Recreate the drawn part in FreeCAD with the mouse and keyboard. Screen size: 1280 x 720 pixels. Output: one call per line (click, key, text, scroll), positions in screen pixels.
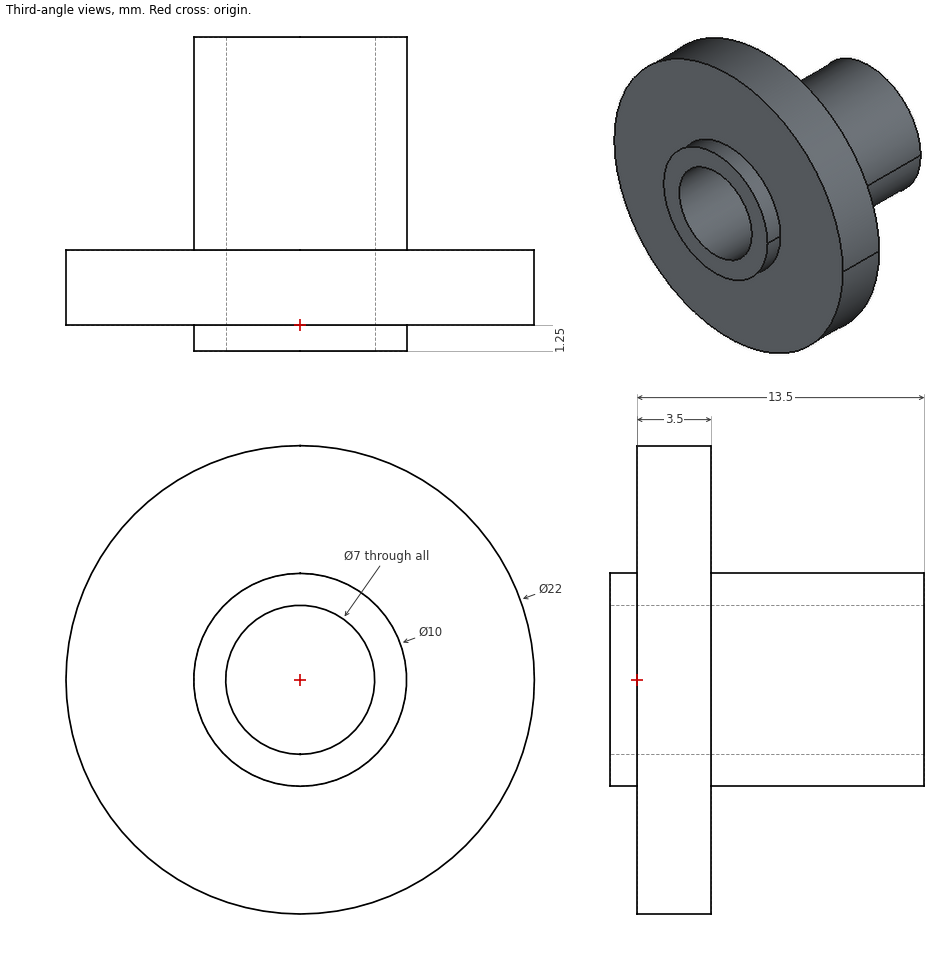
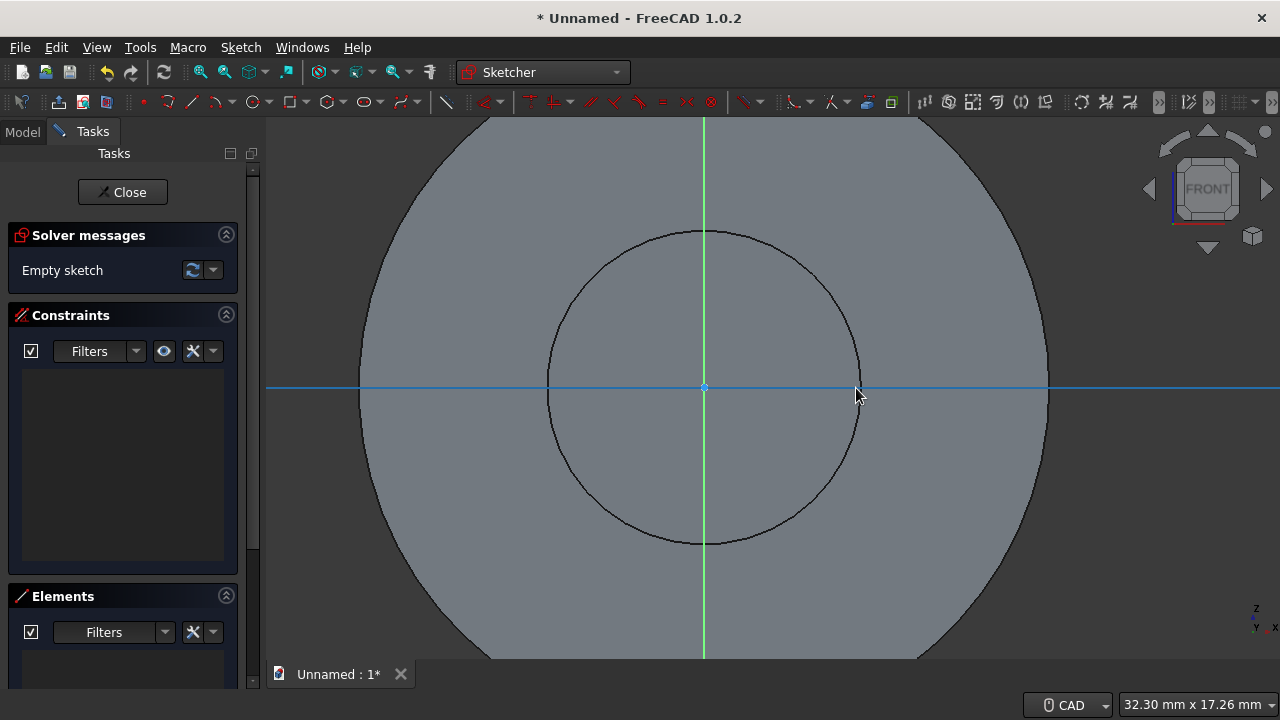
key(g)
key(c)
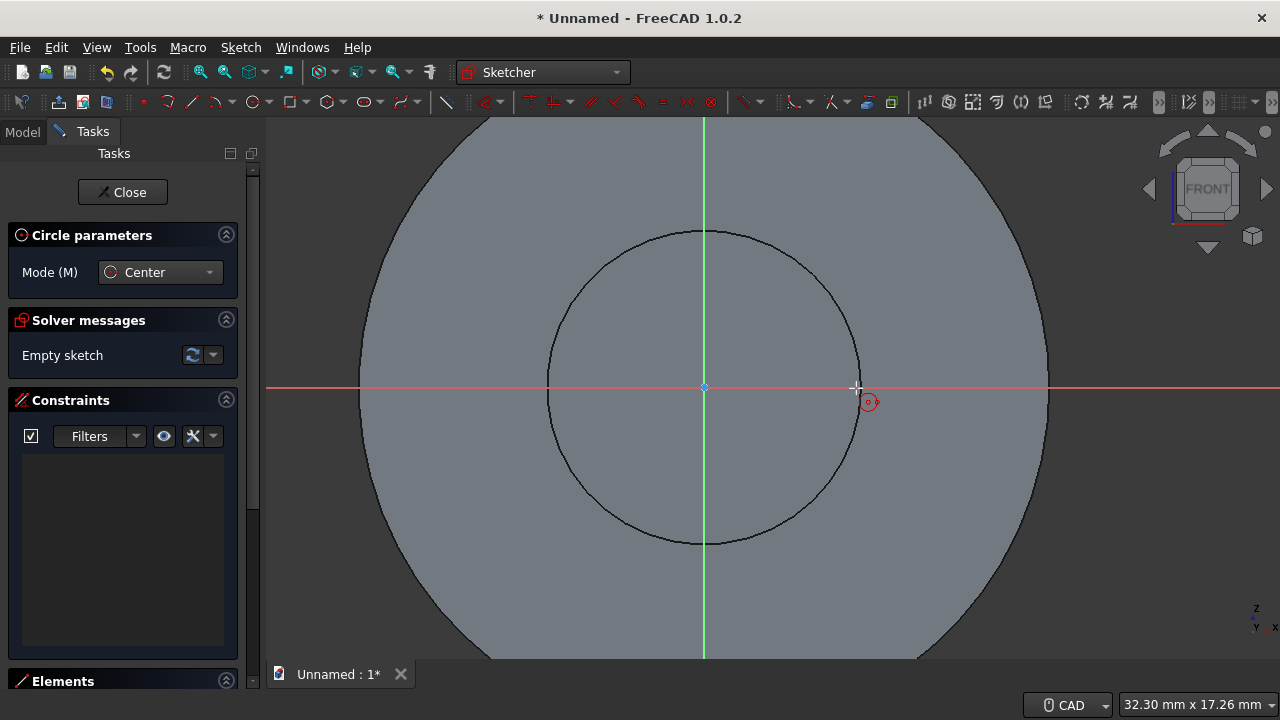
click(704, 388)
move(815, 277)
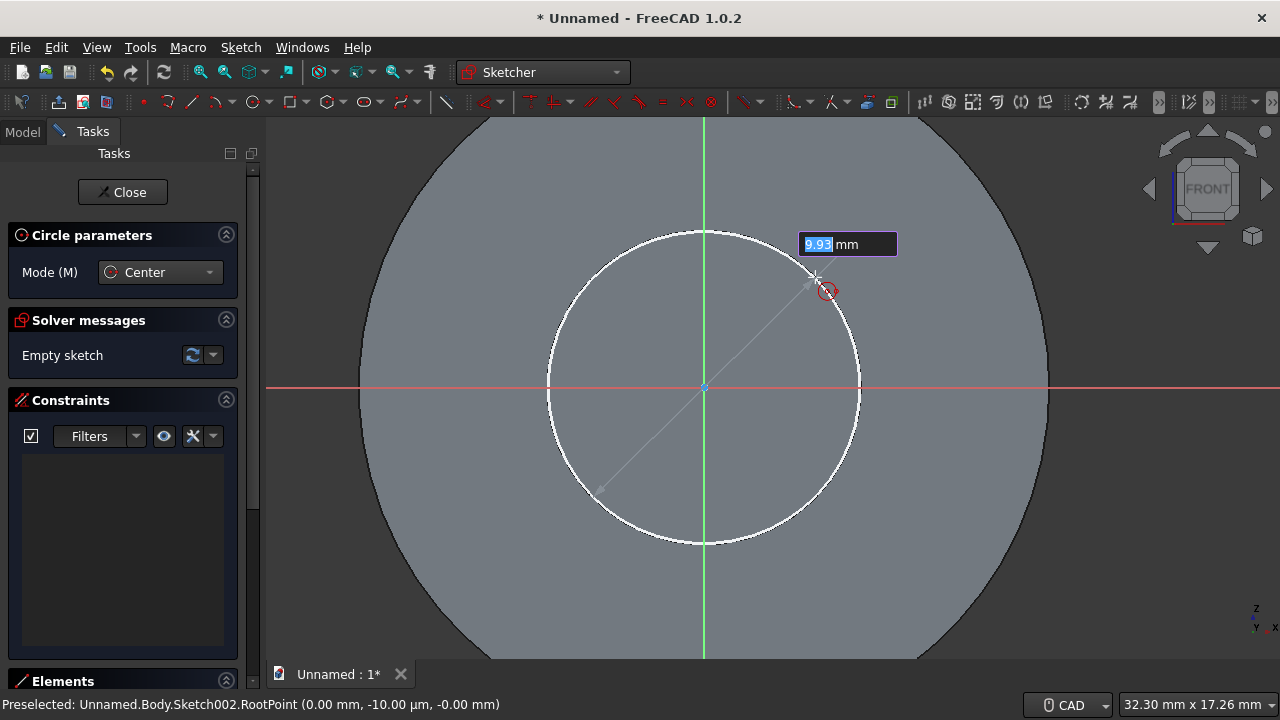
text(10)
key(Return)
key(Escape)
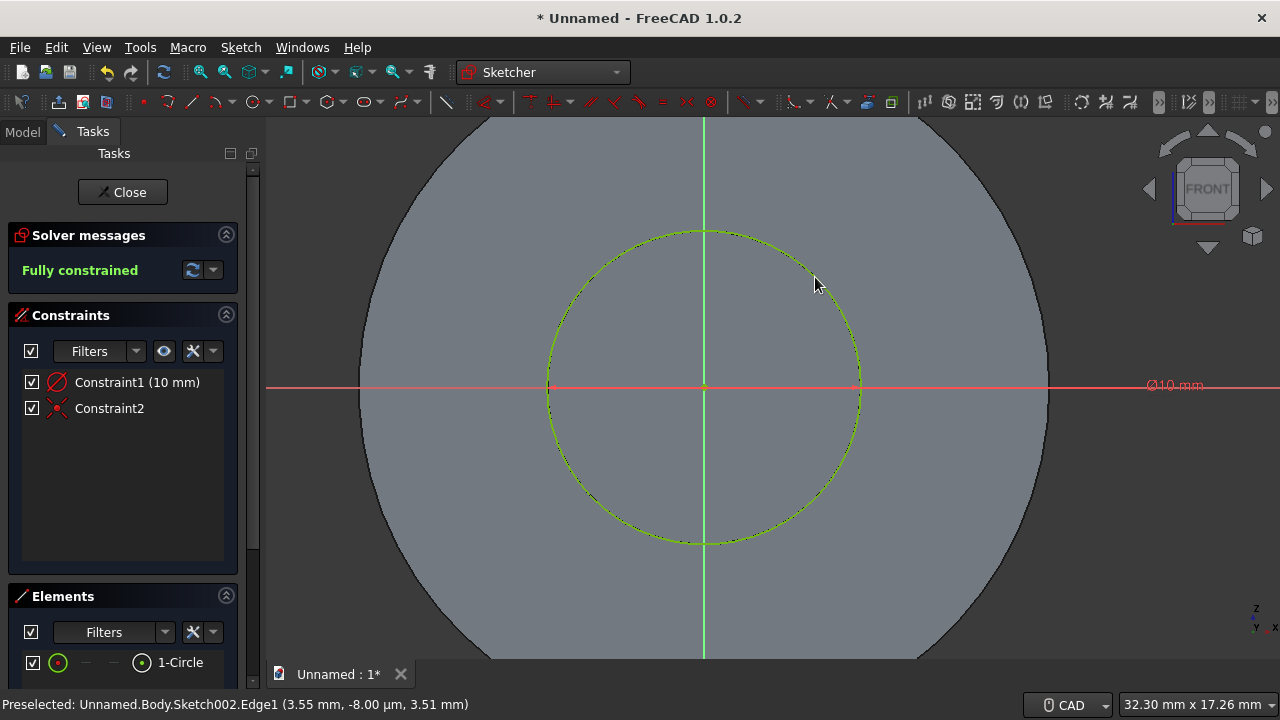
click(123, 192)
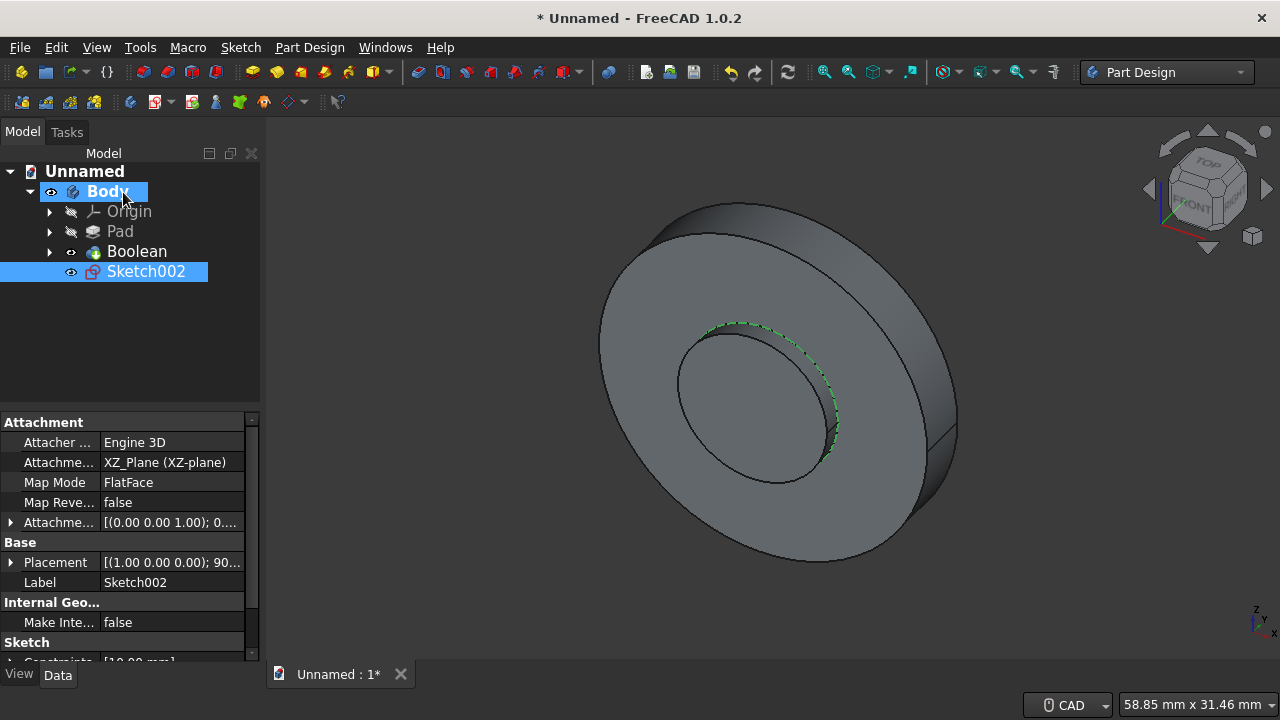
click(254, 72)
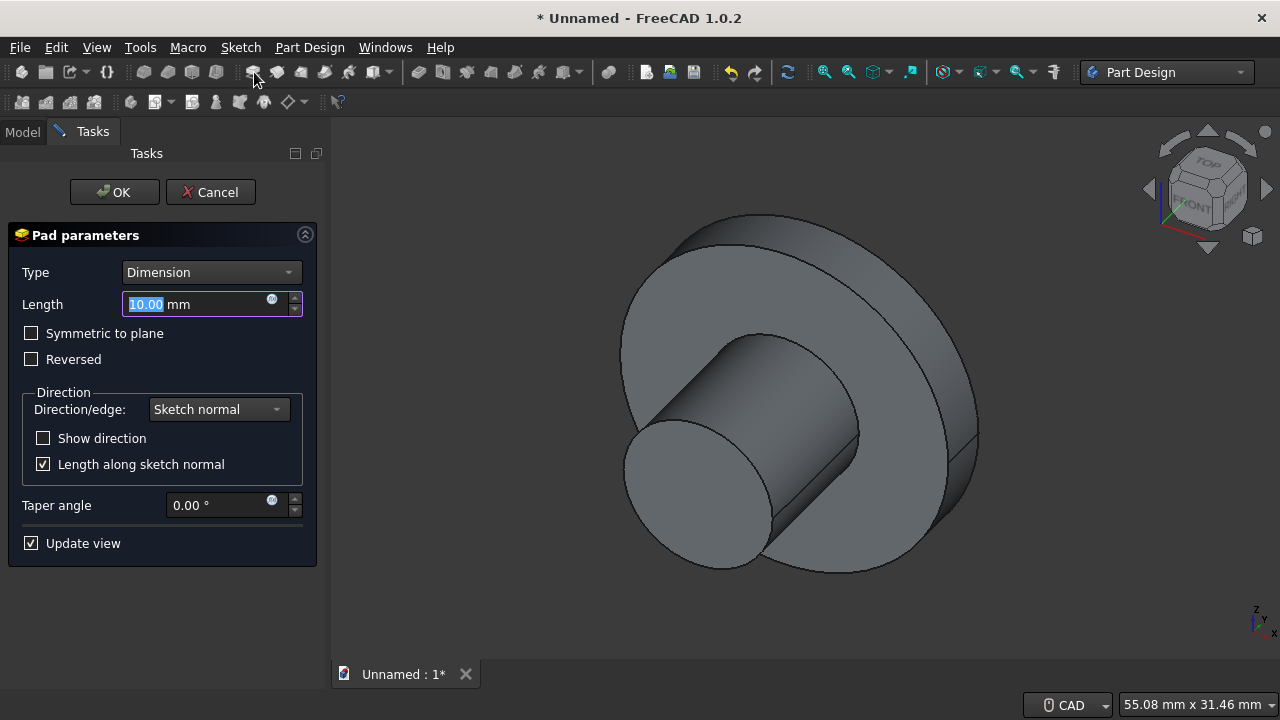
text(13.5)
key(Tab)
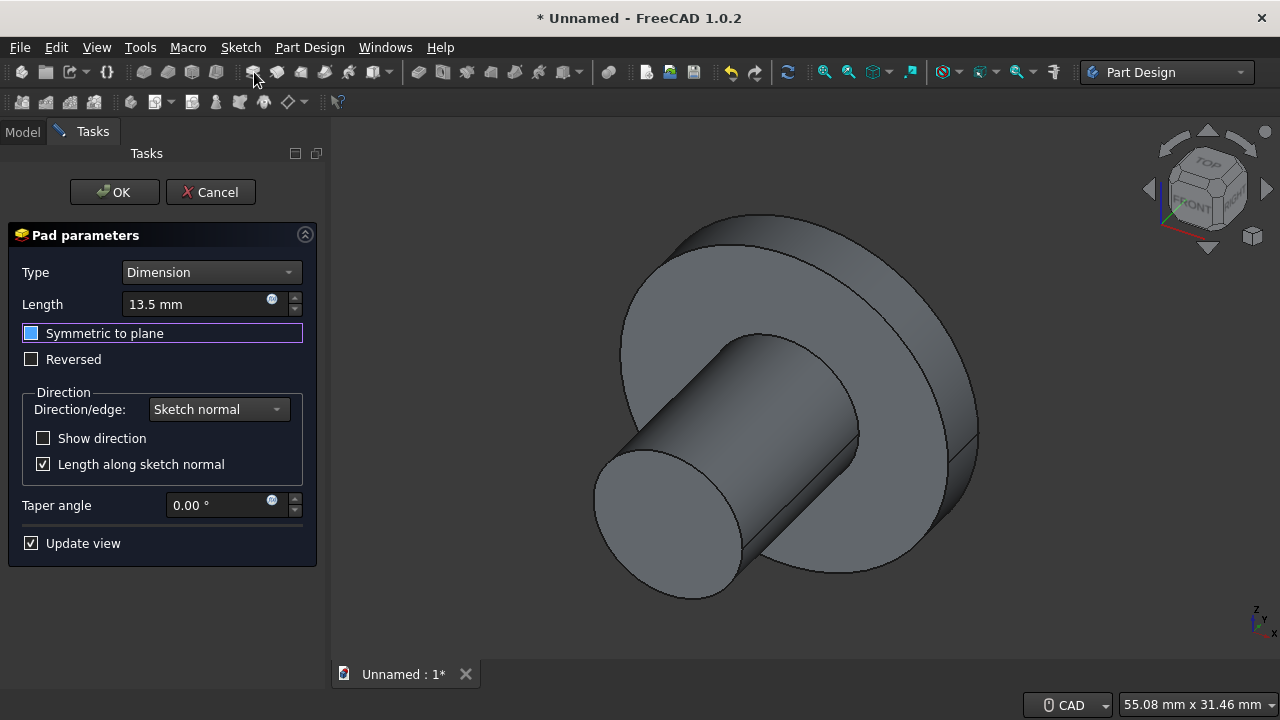
click(30, 359)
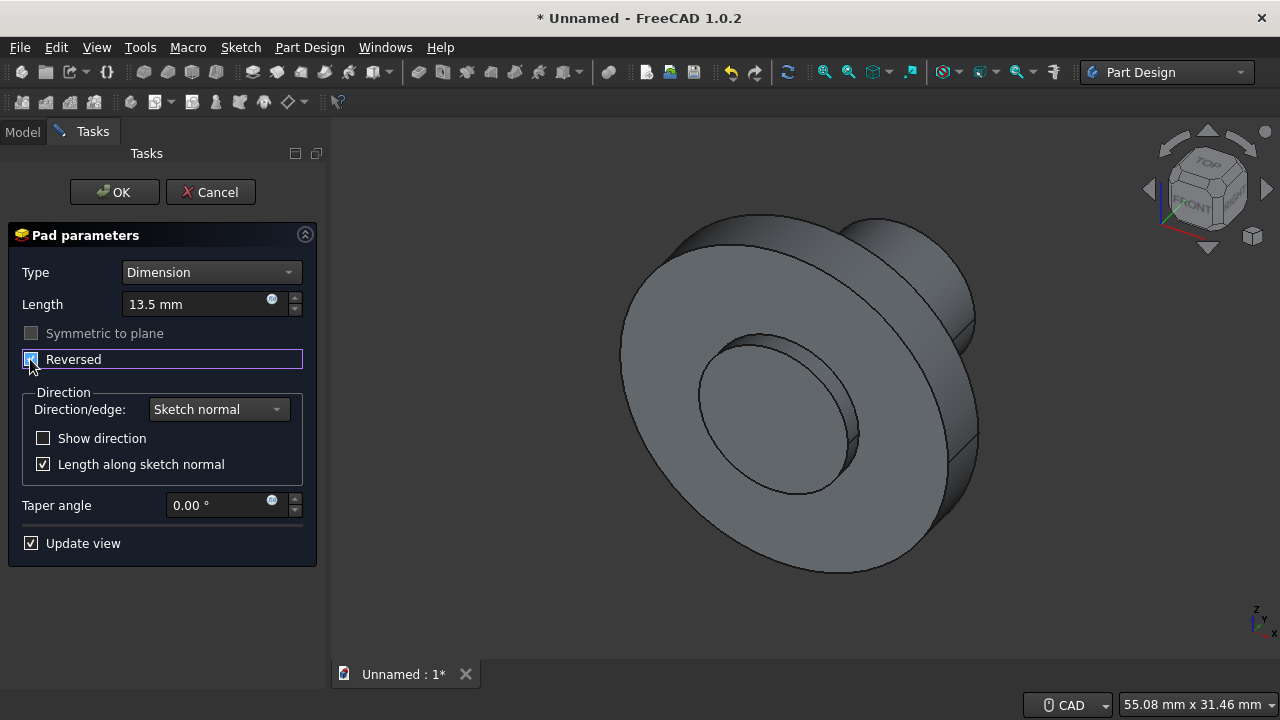
click(115, 192)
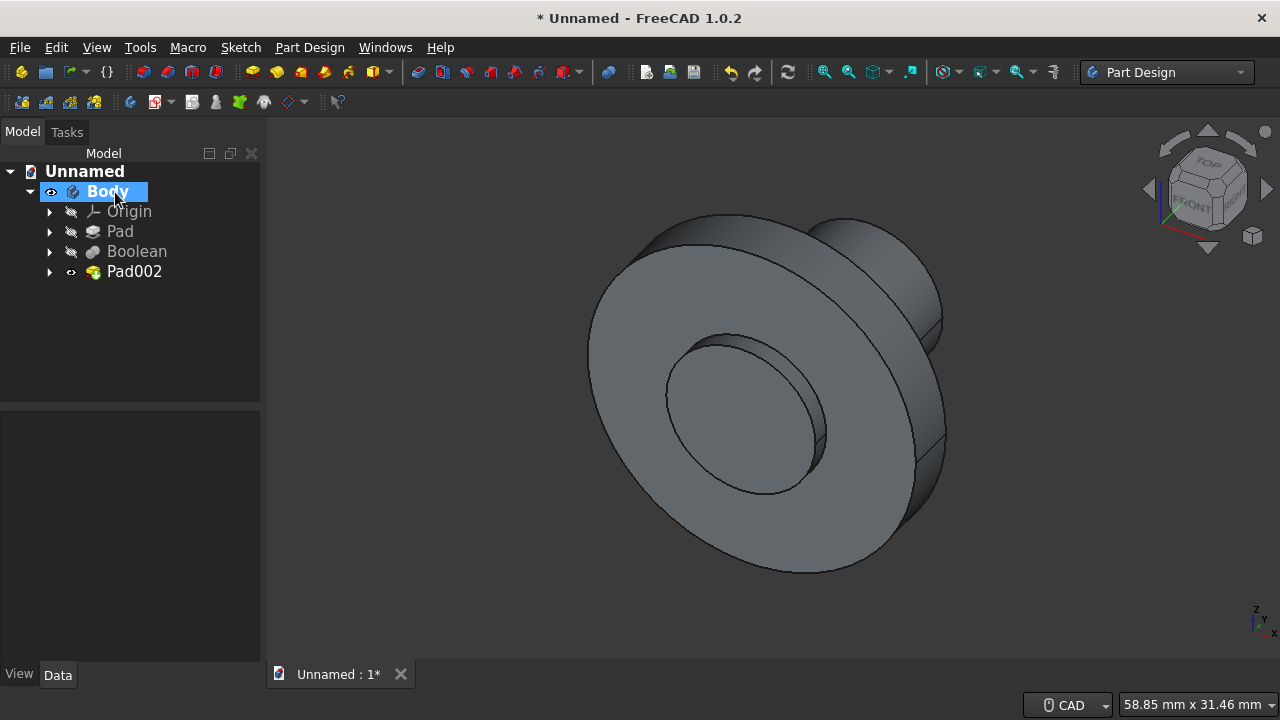
click(826, 72)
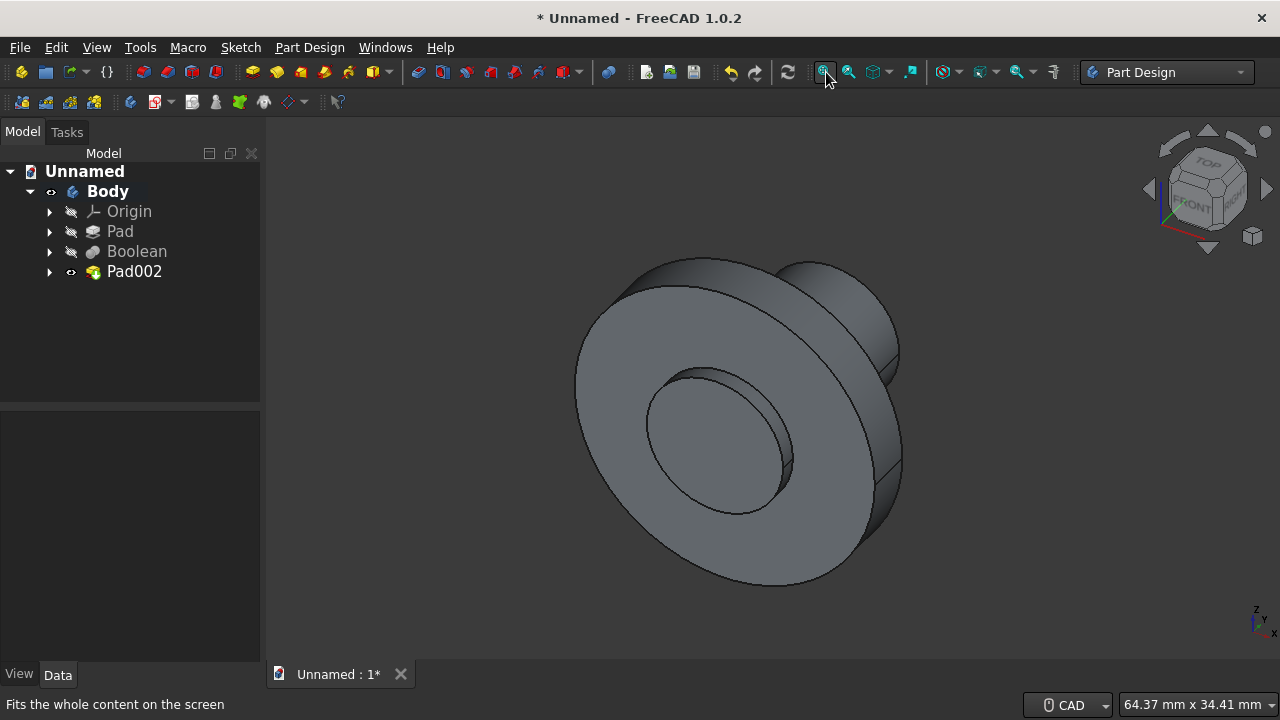
key(4)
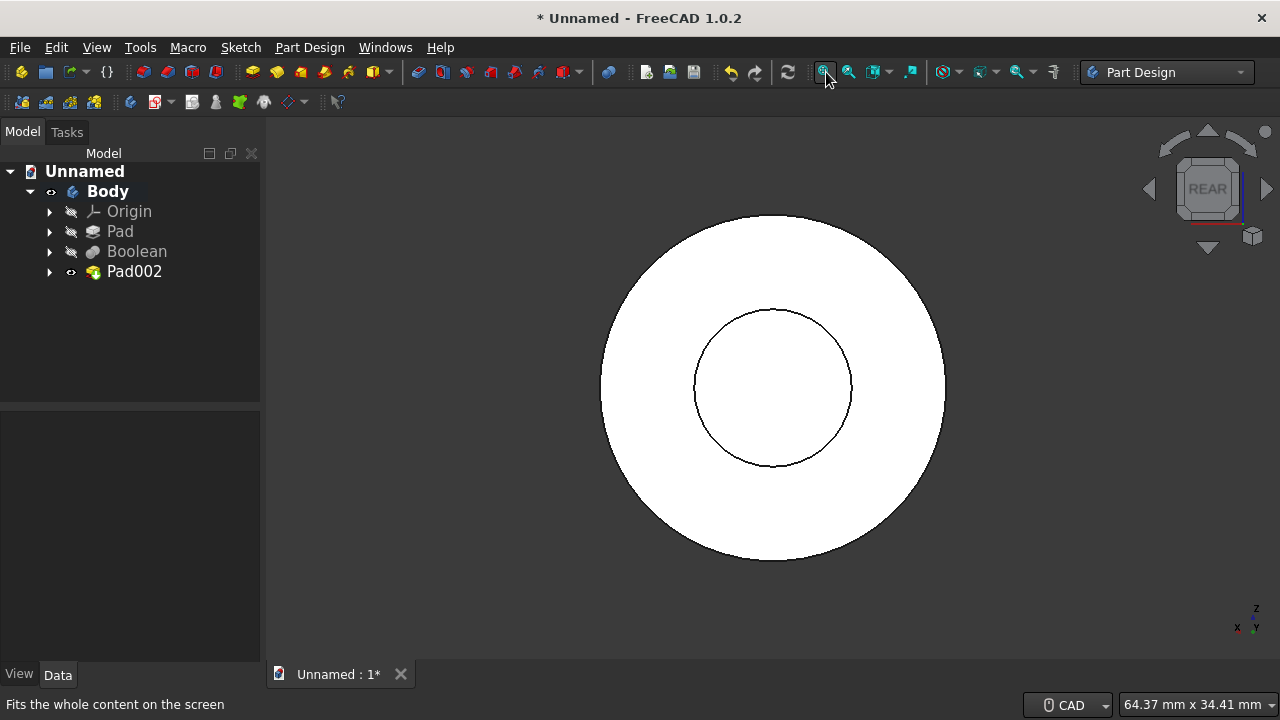
click(773, 387)